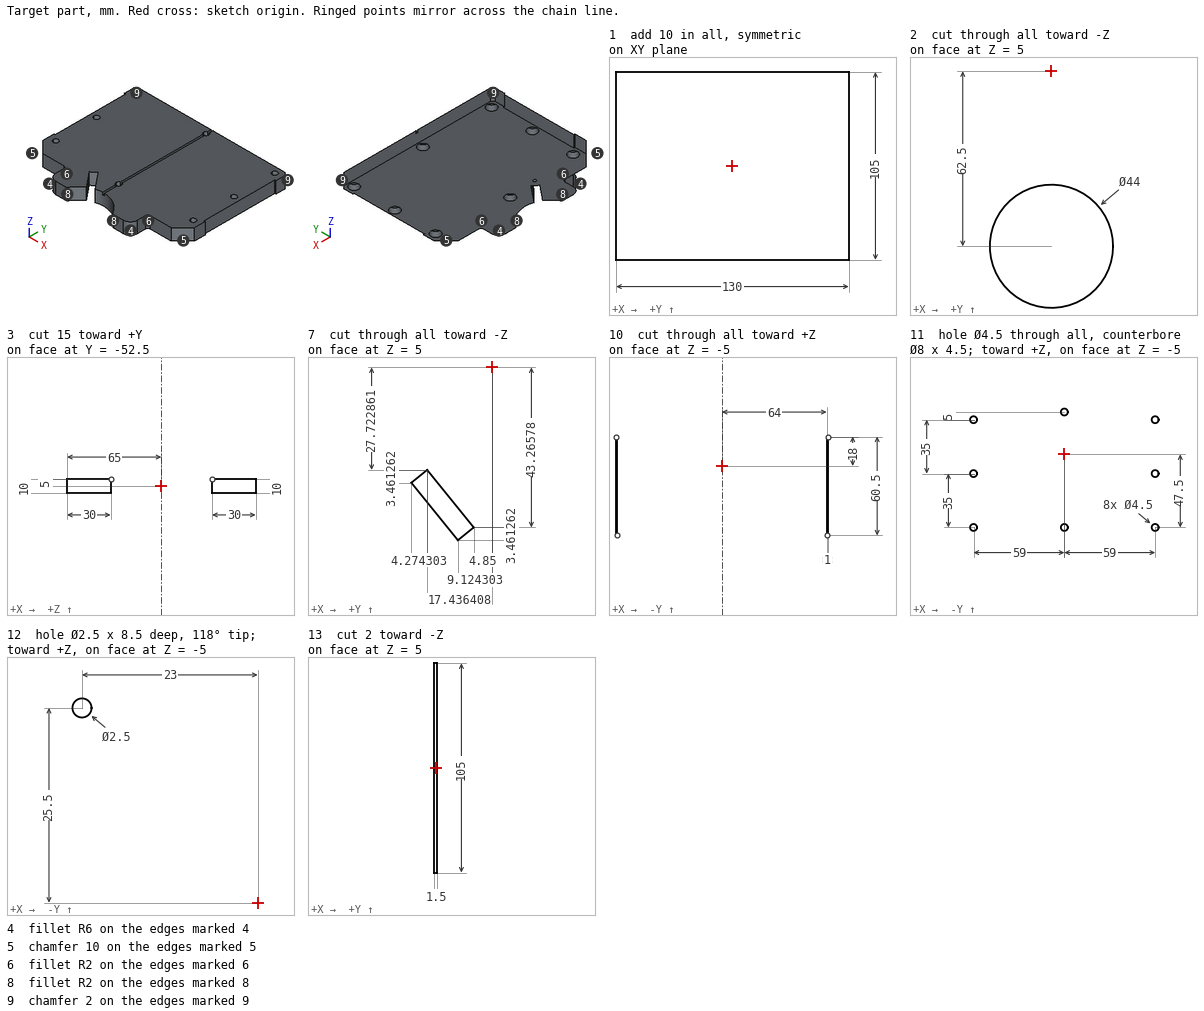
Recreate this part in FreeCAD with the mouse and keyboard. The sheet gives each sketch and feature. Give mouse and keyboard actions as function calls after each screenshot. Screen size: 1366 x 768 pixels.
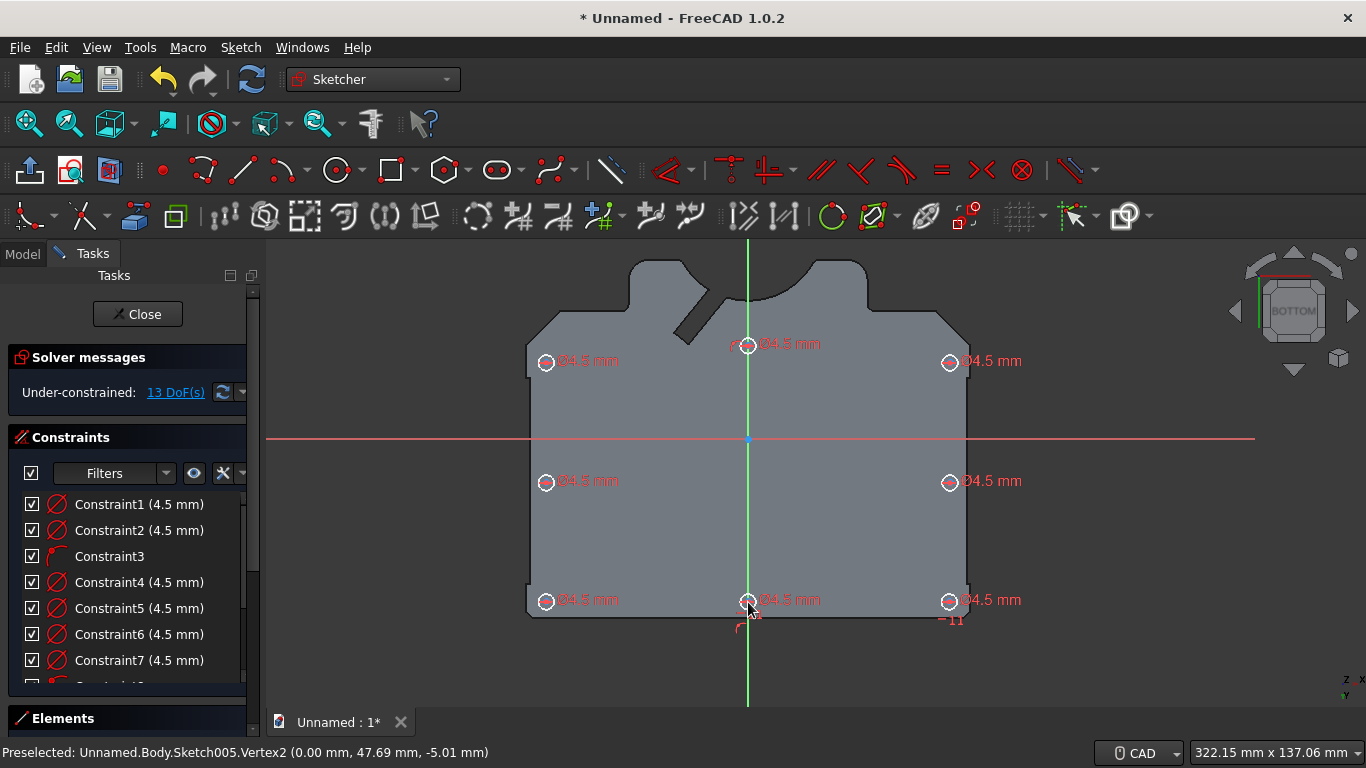
click(748, 602)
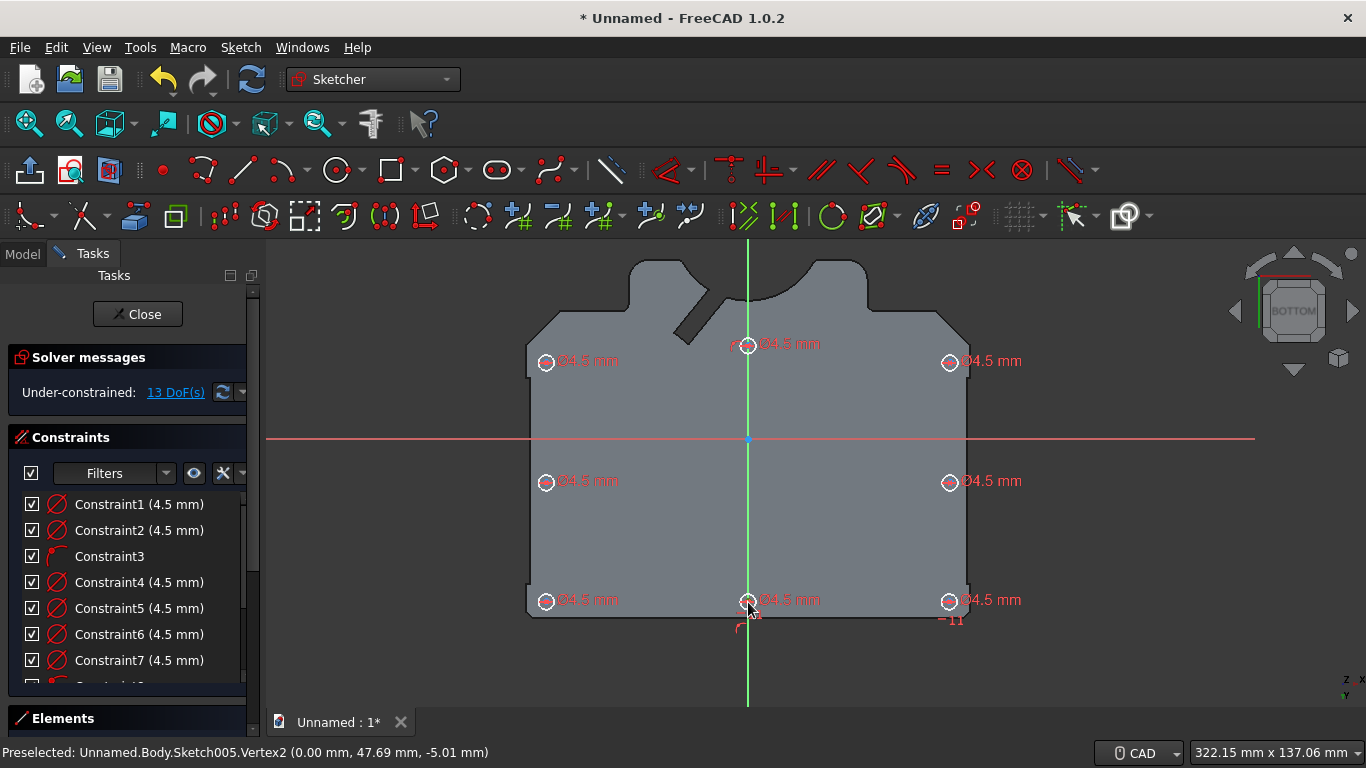
click(546, 602)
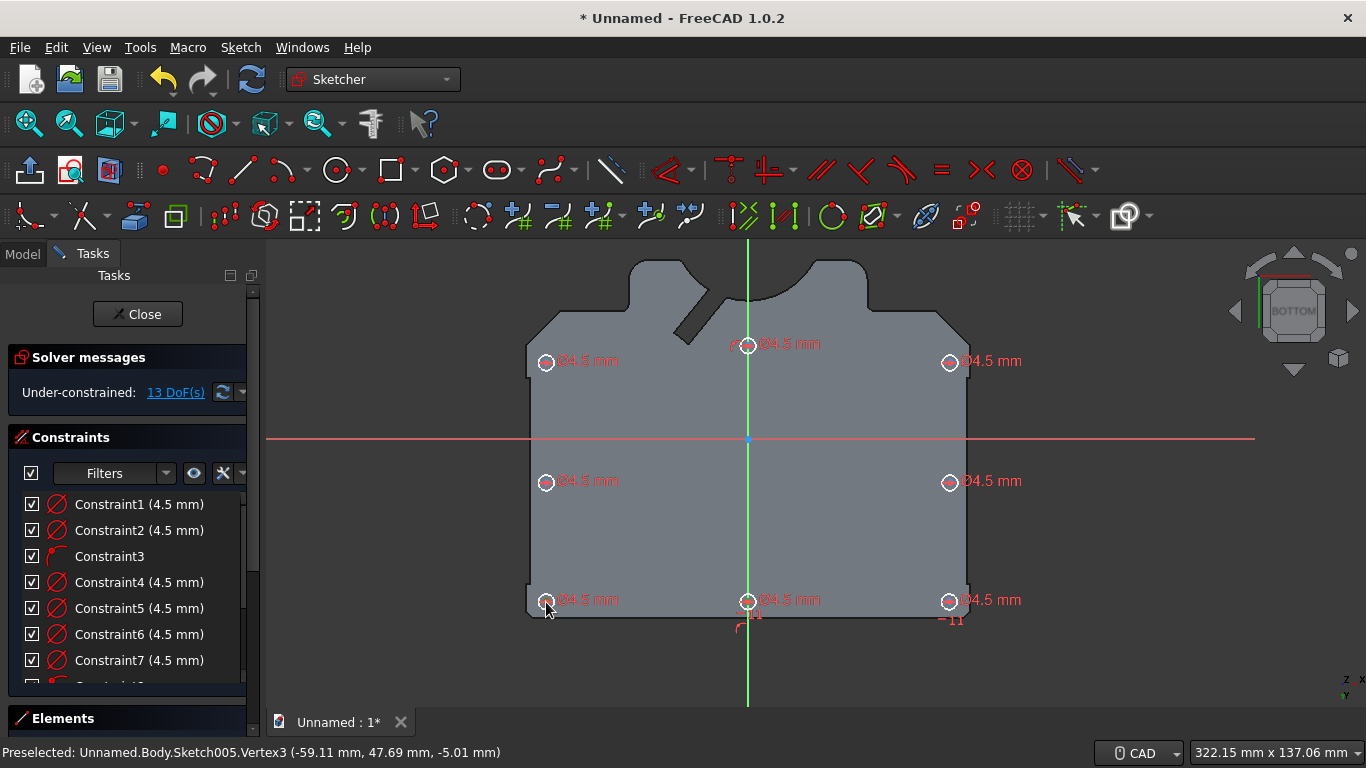
click(796, 170)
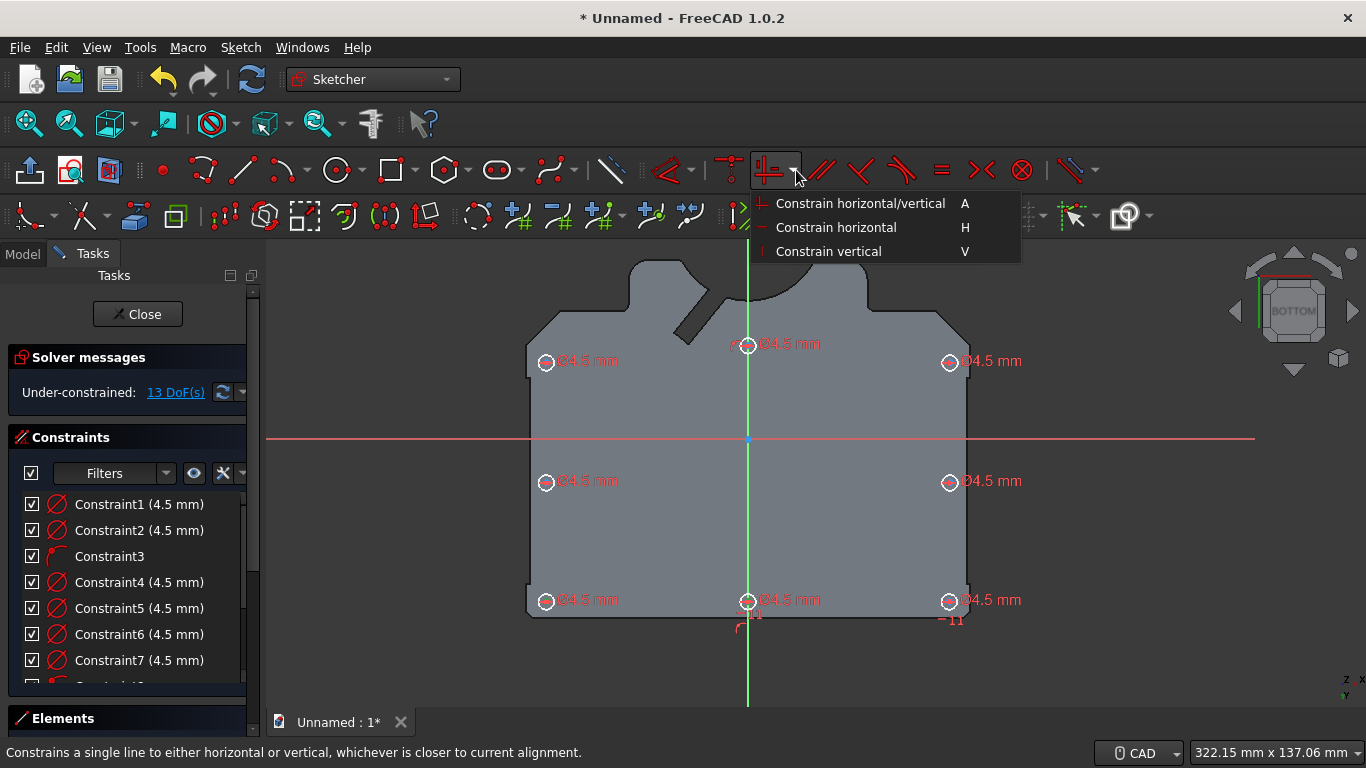
click(886, 227)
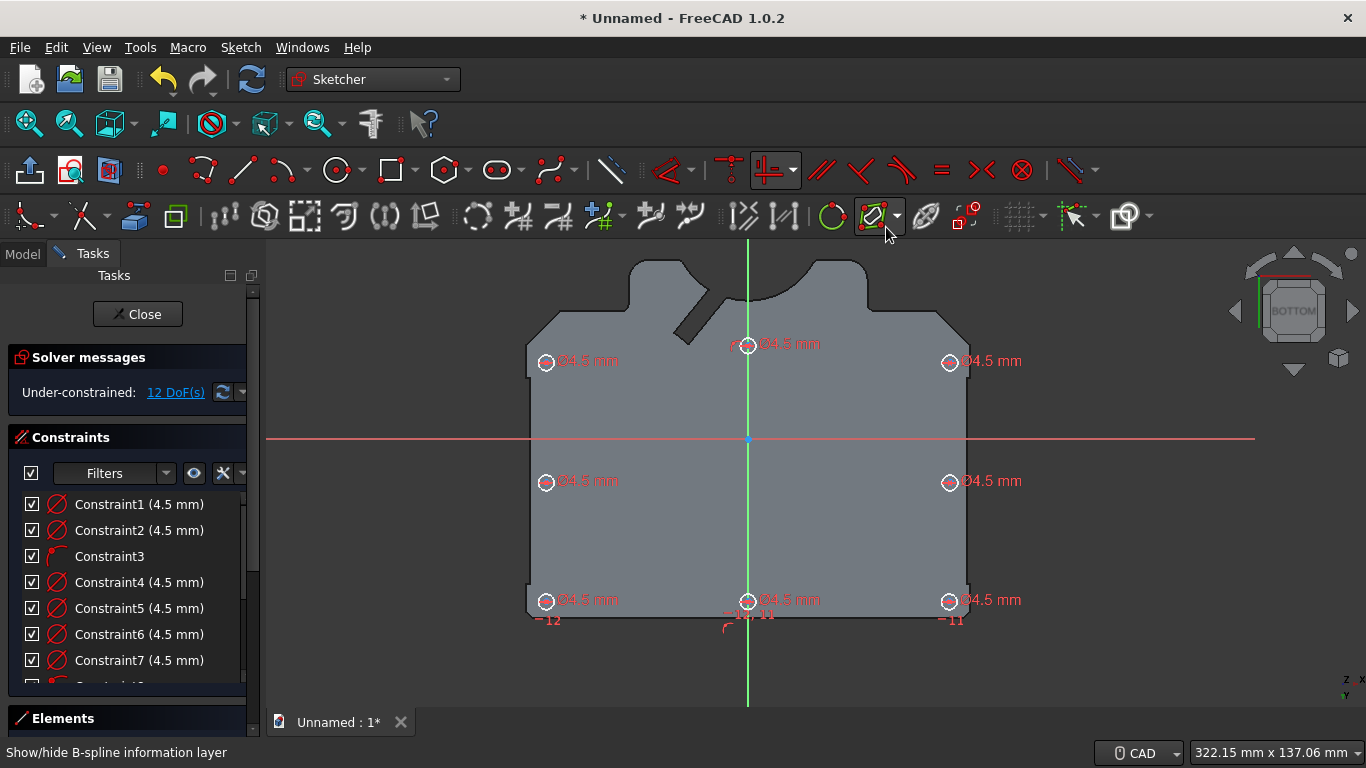
click(546, 602)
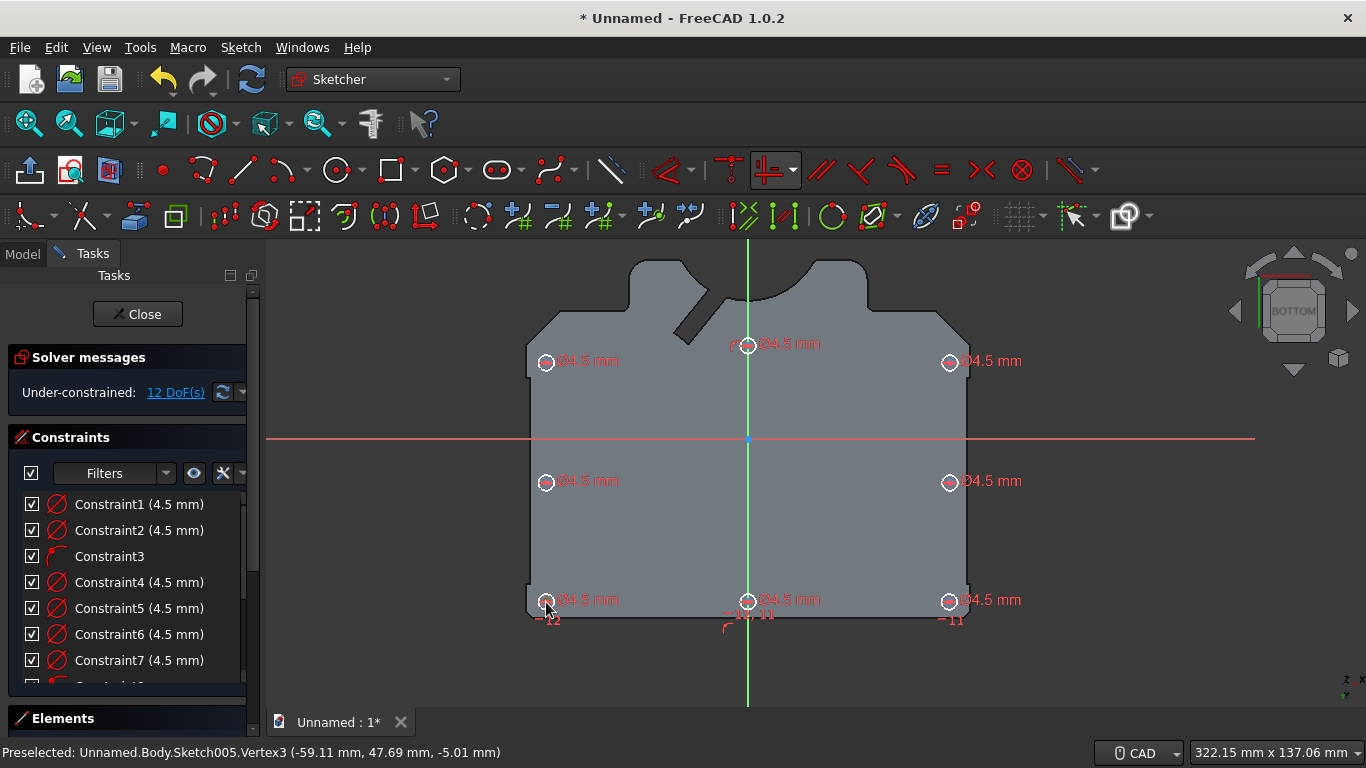
click(546, 483)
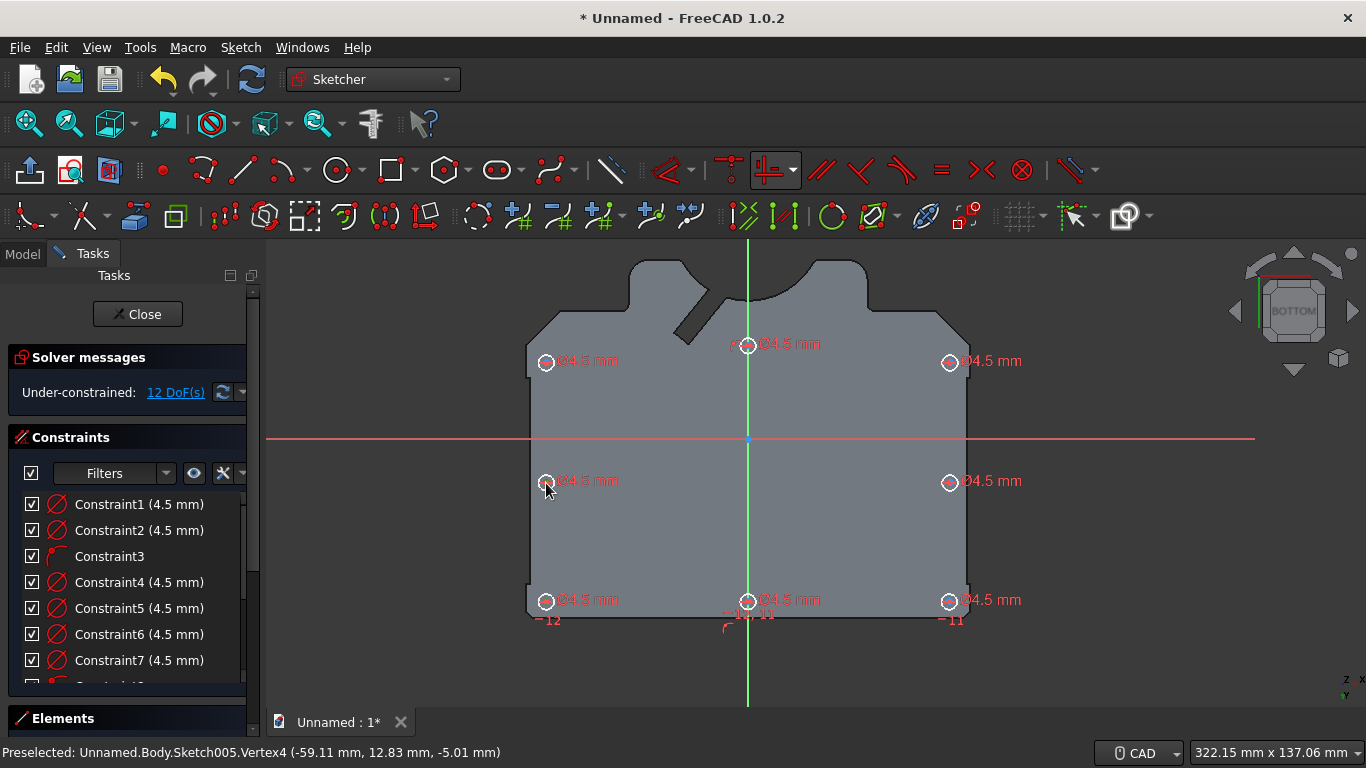
key(v)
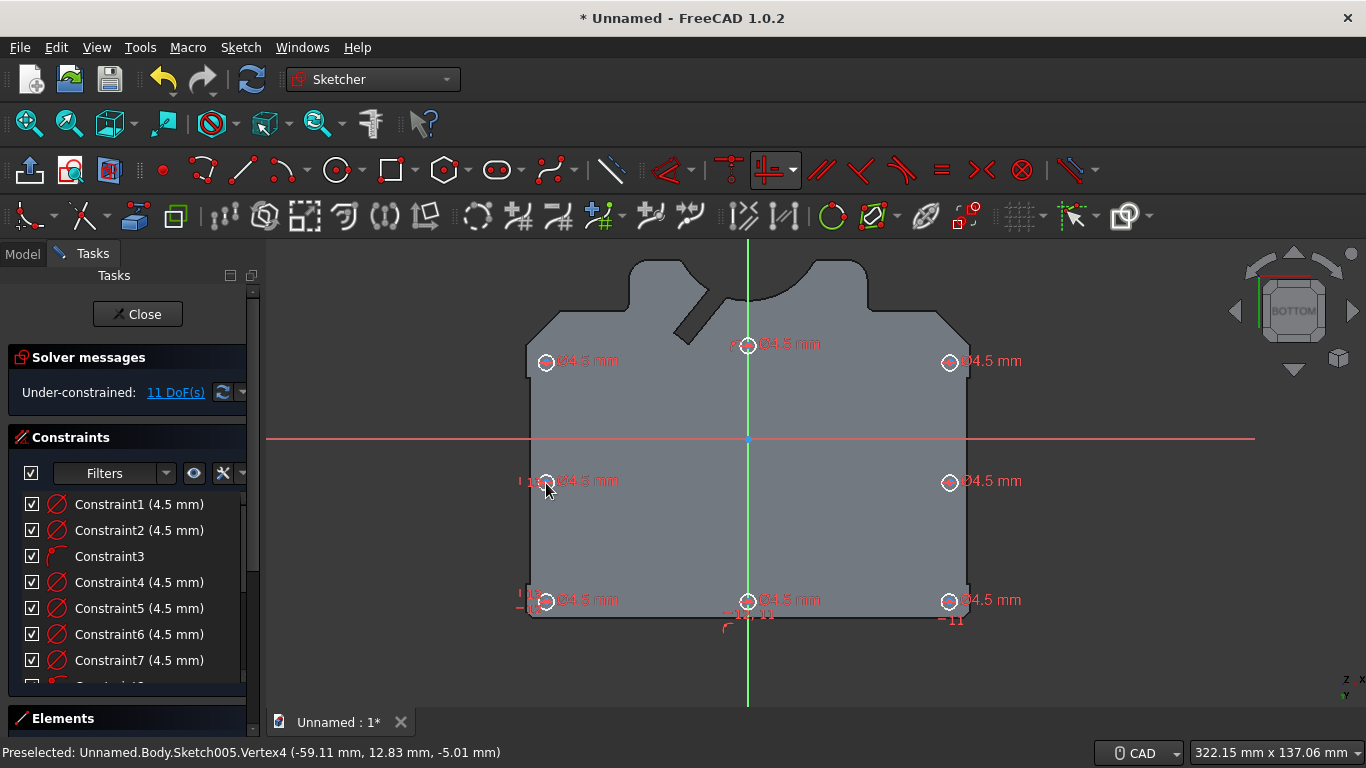
click(546, 483)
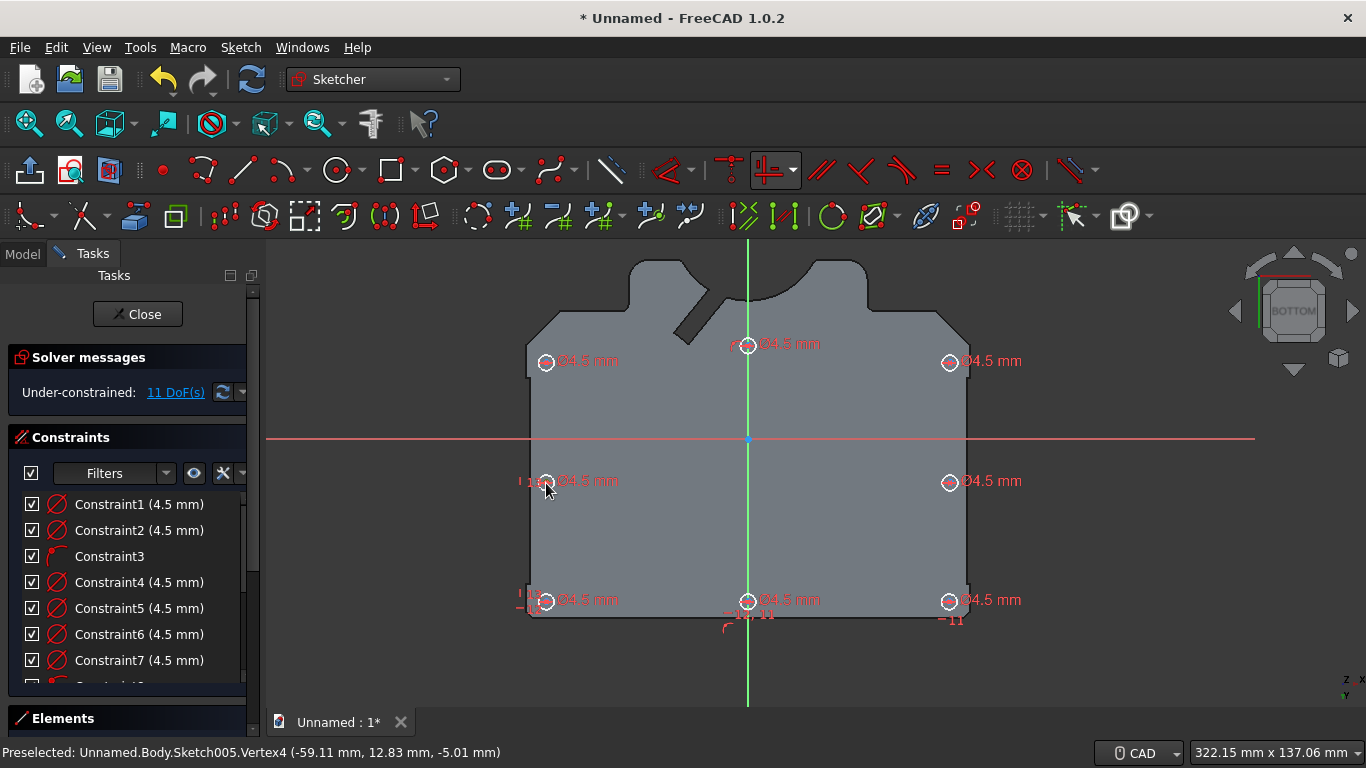
click(546, 363)